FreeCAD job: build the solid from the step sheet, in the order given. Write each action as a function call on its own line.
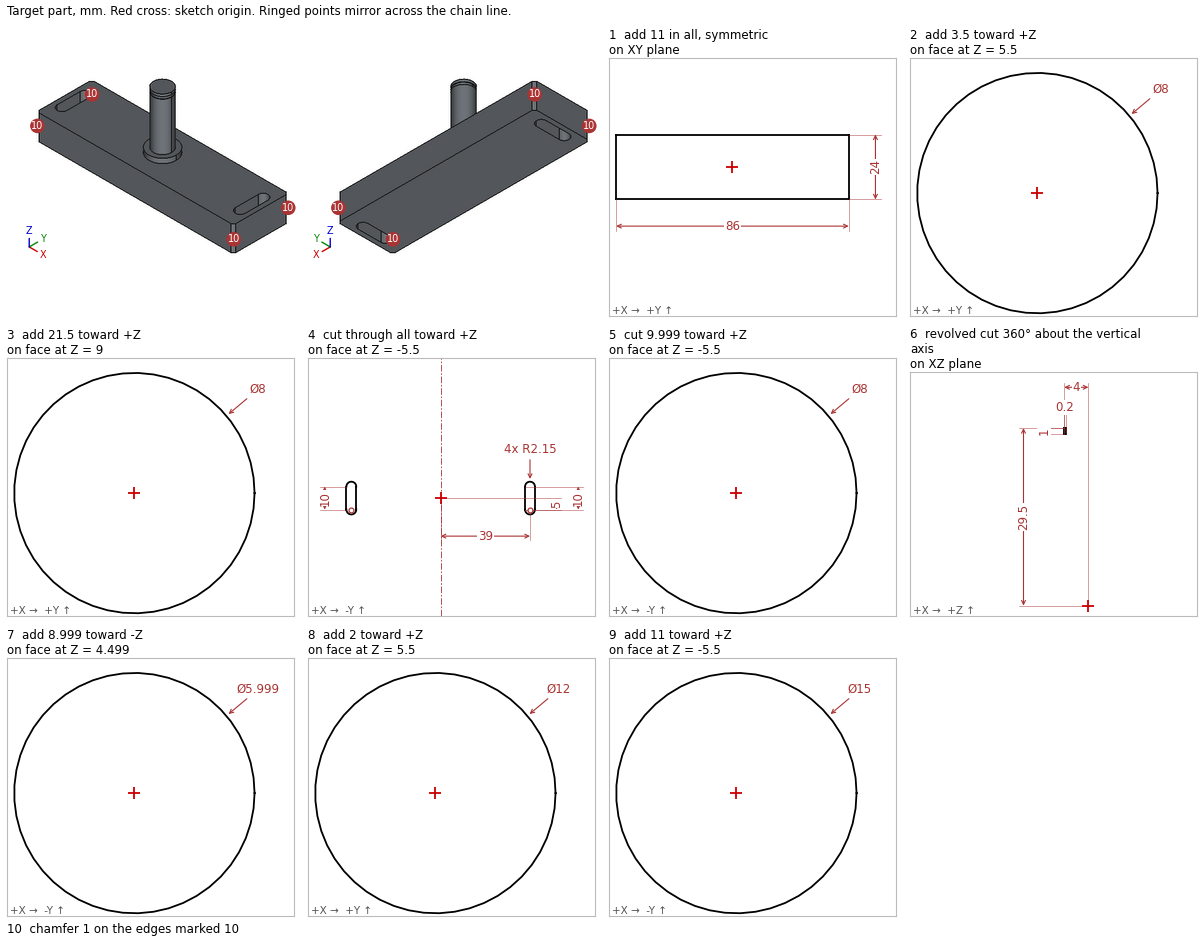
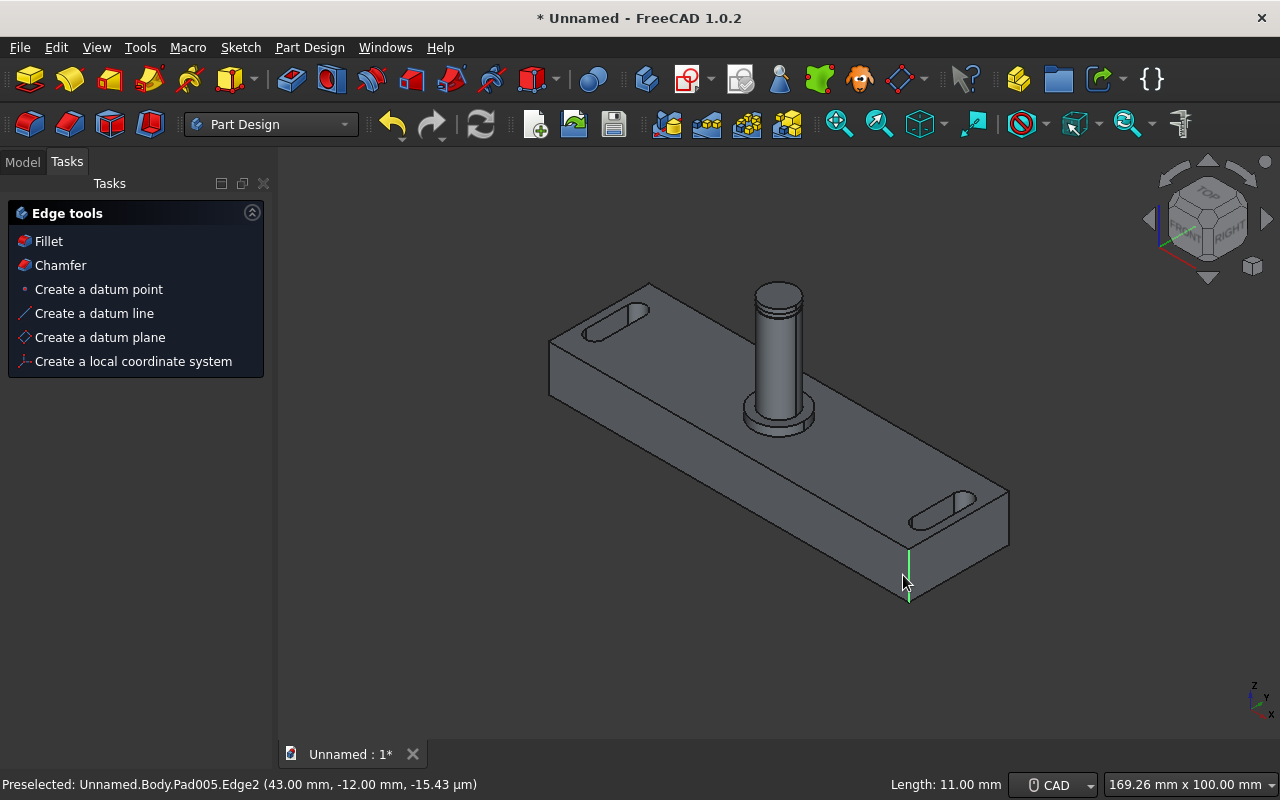
key(2)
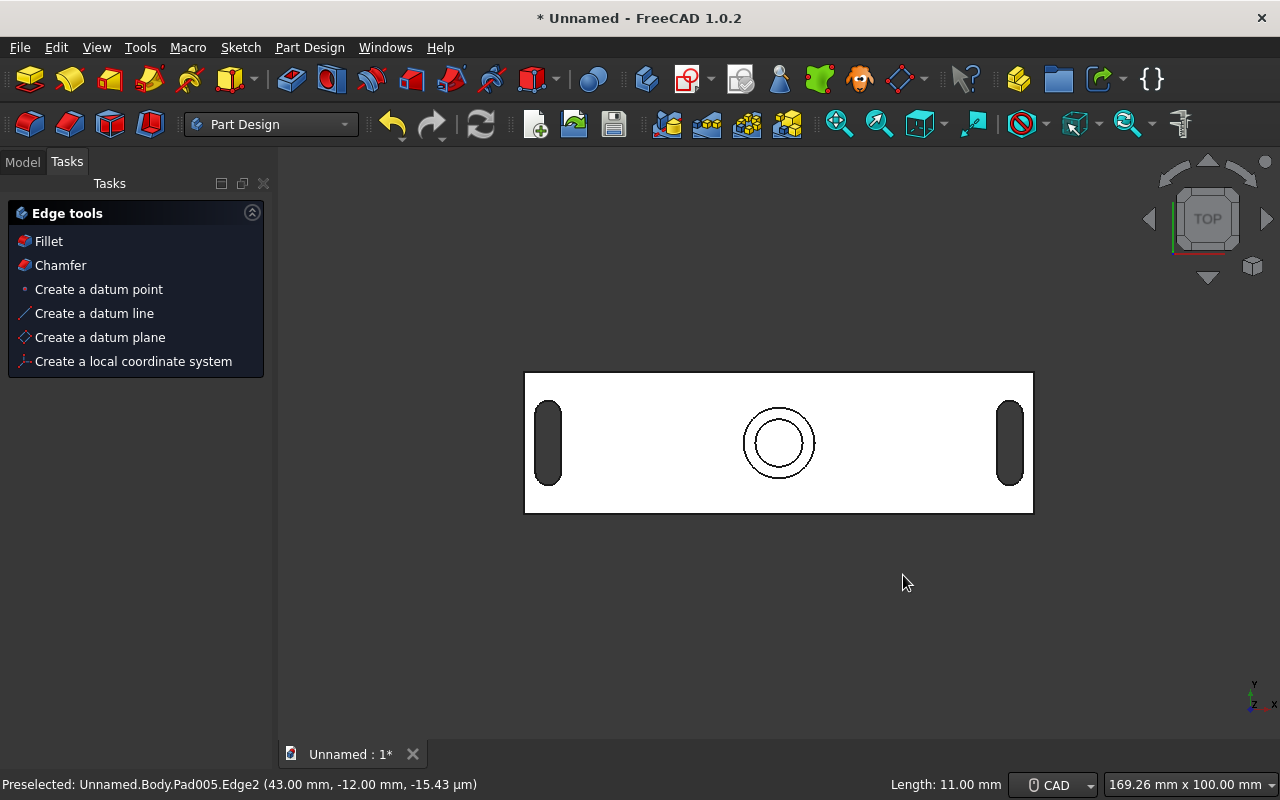
key(1)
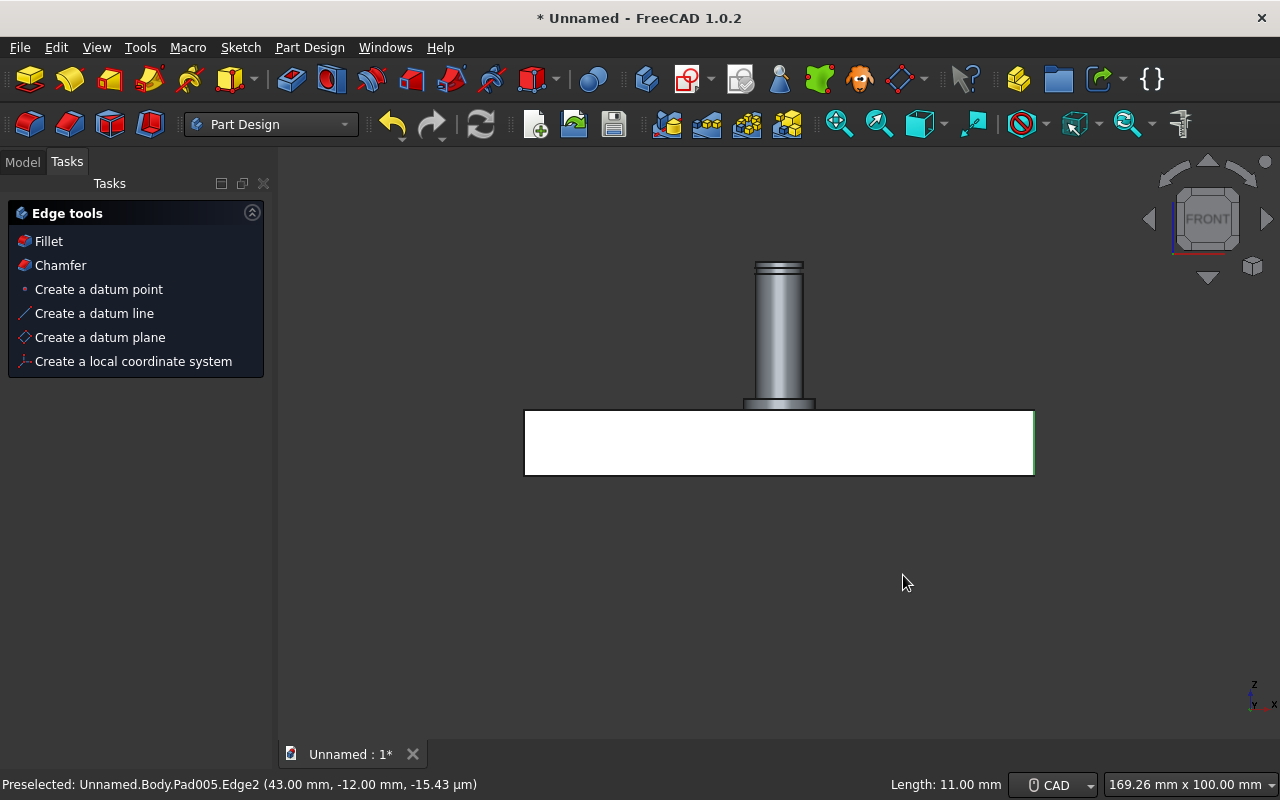
click(524, 442, ctrl)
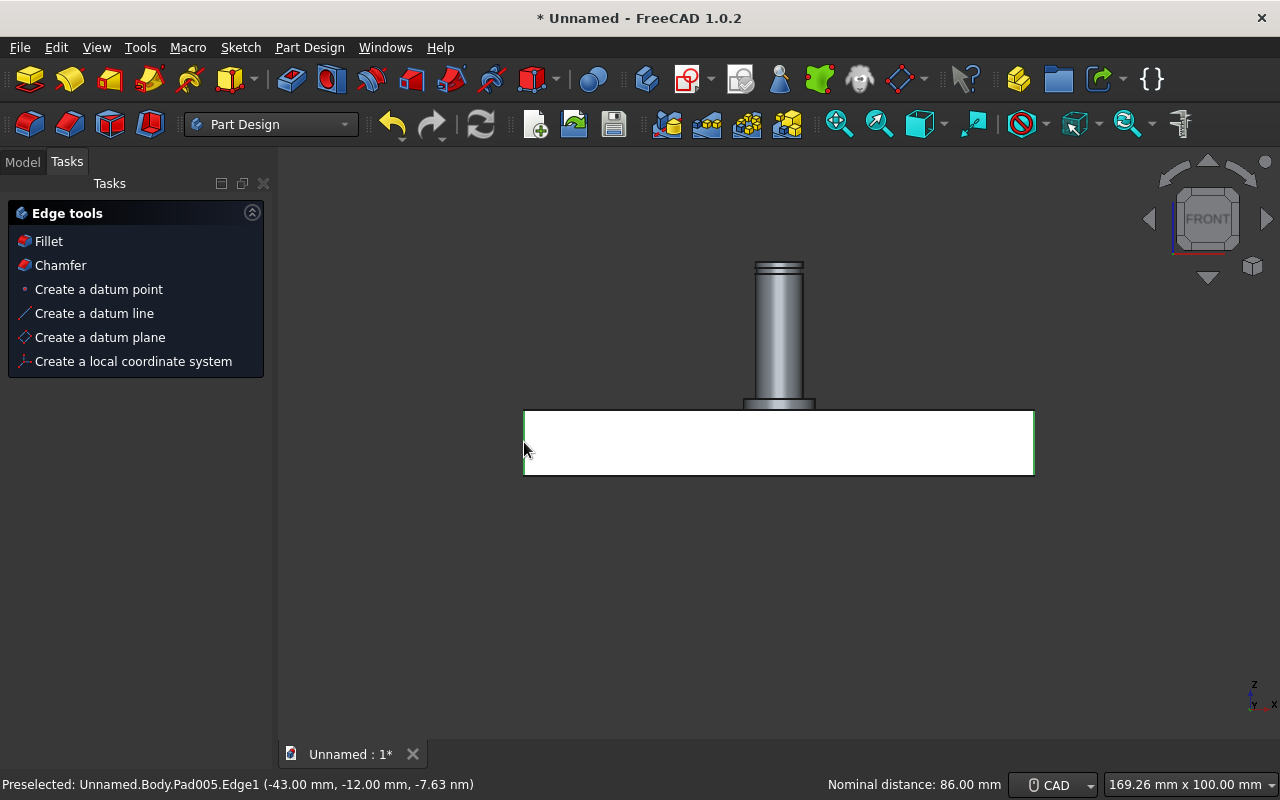
key(3)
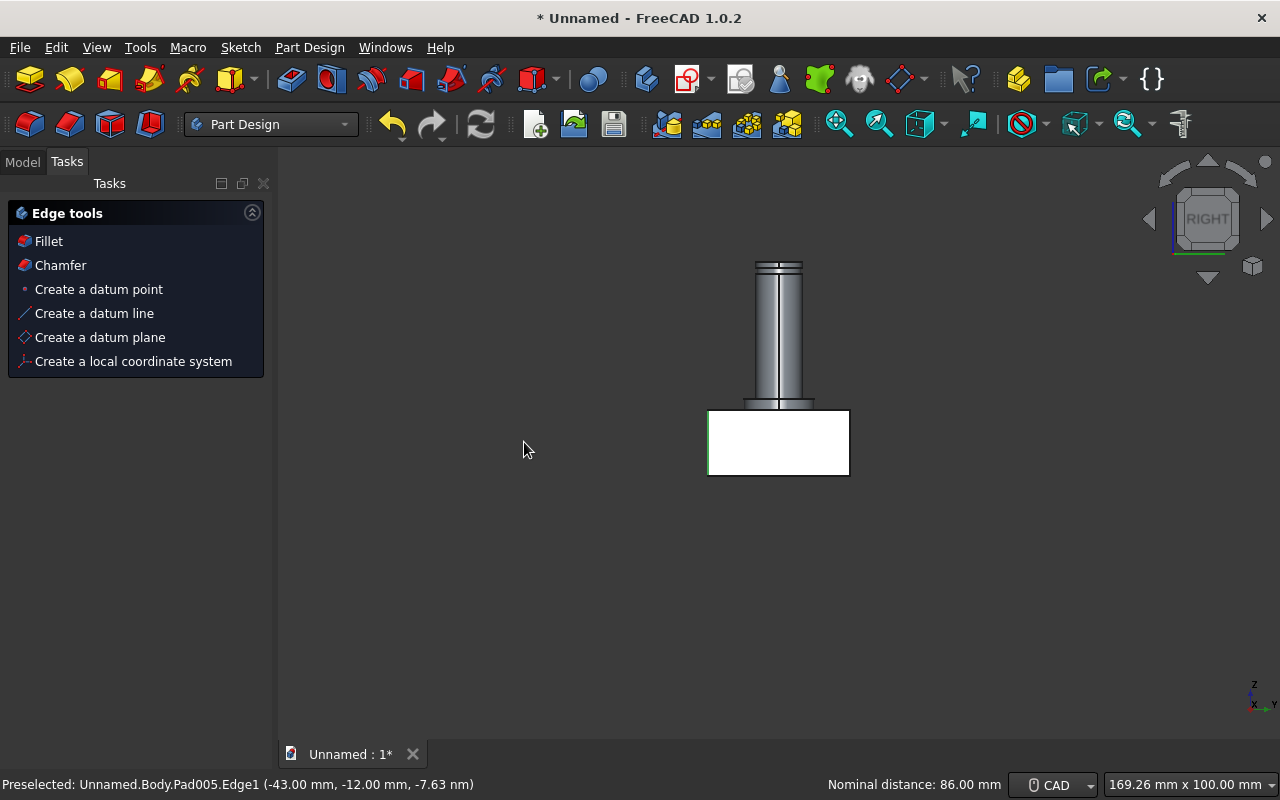
click(840, 124)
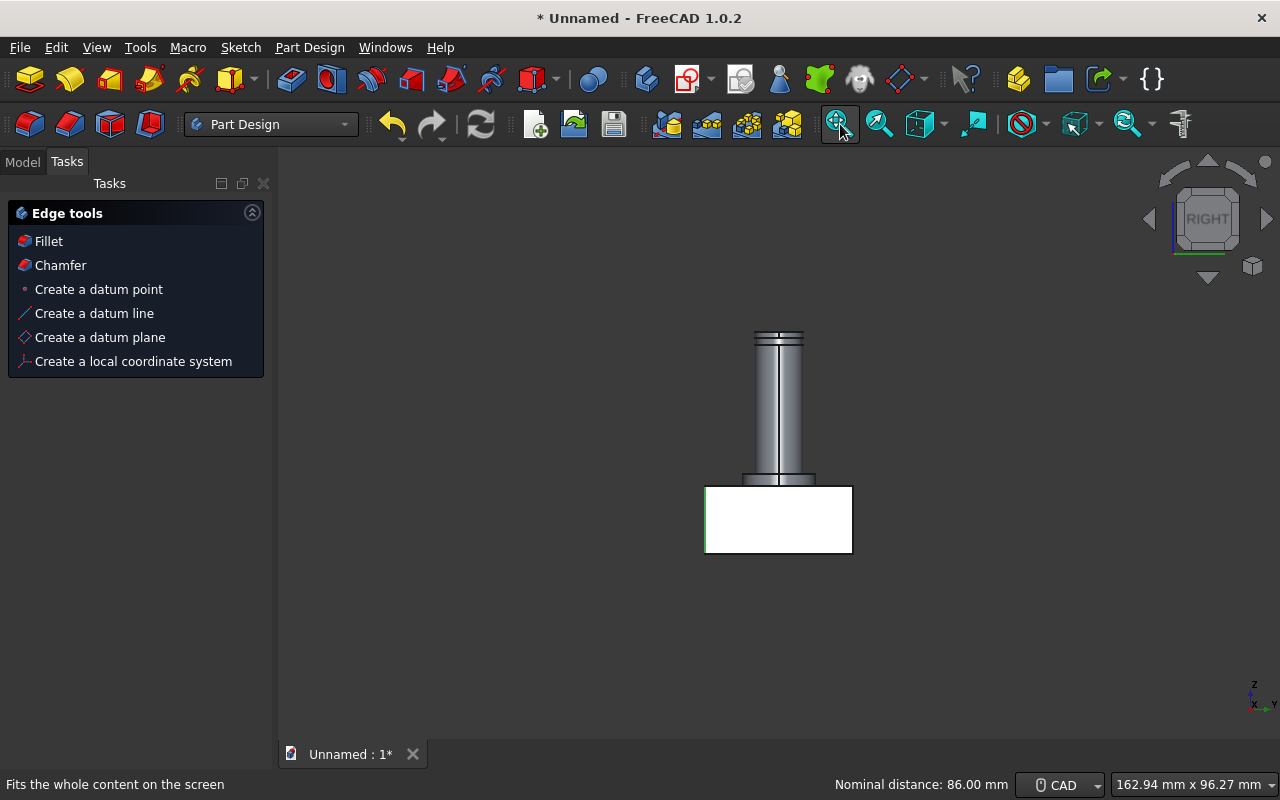
click(853, 519, ctrl)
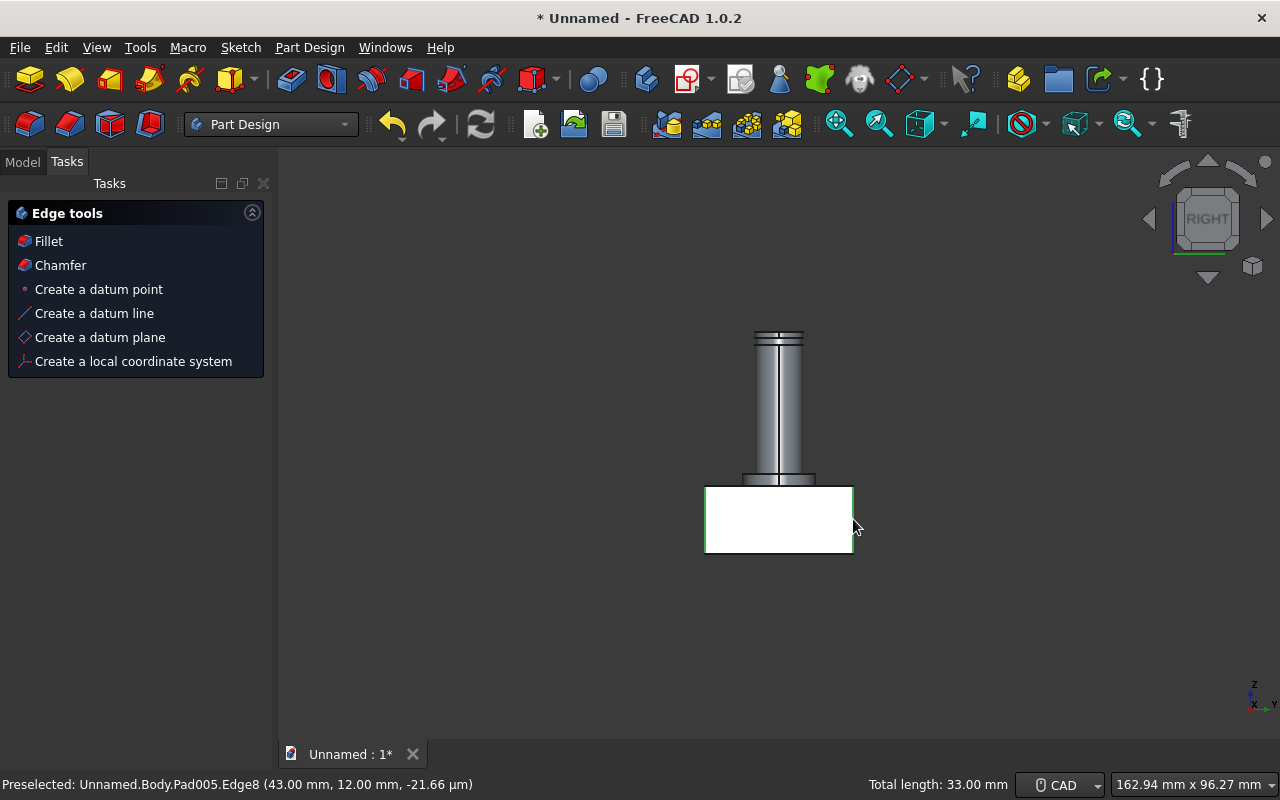
key(5)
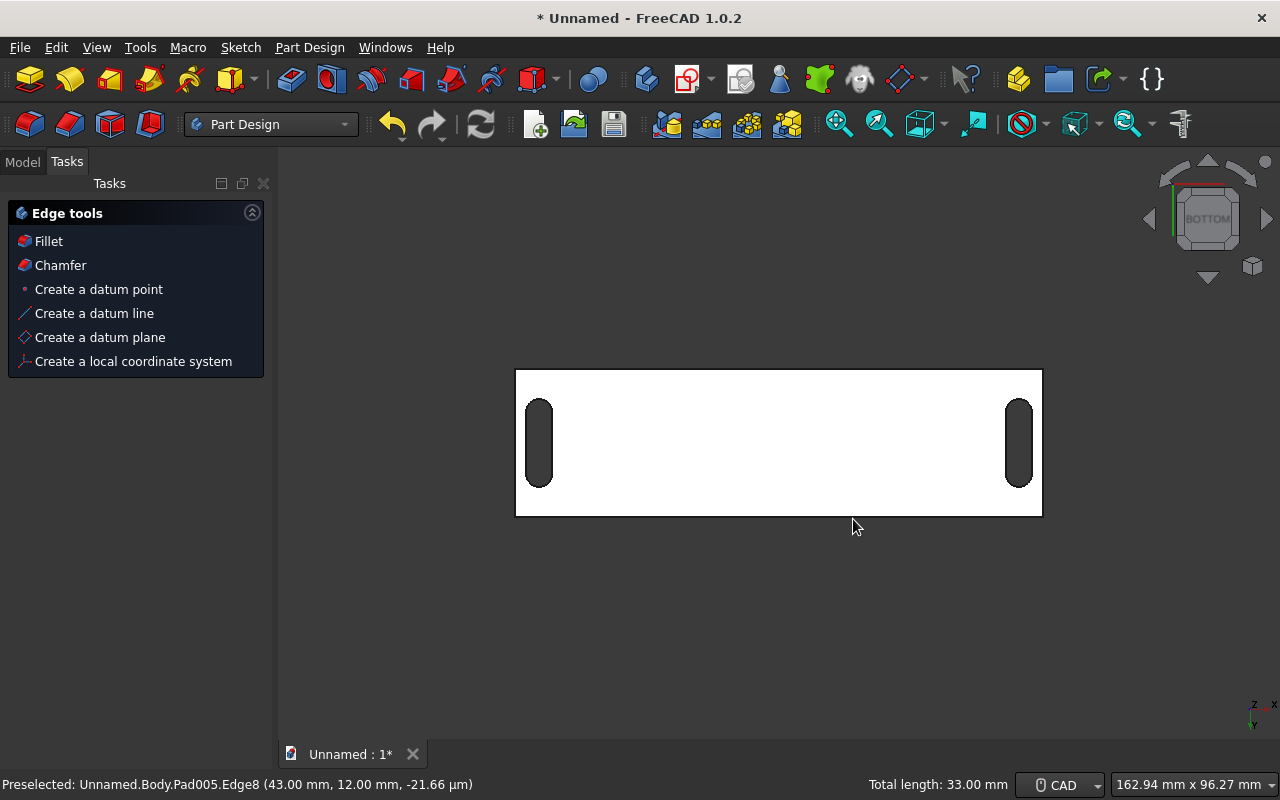
key(4)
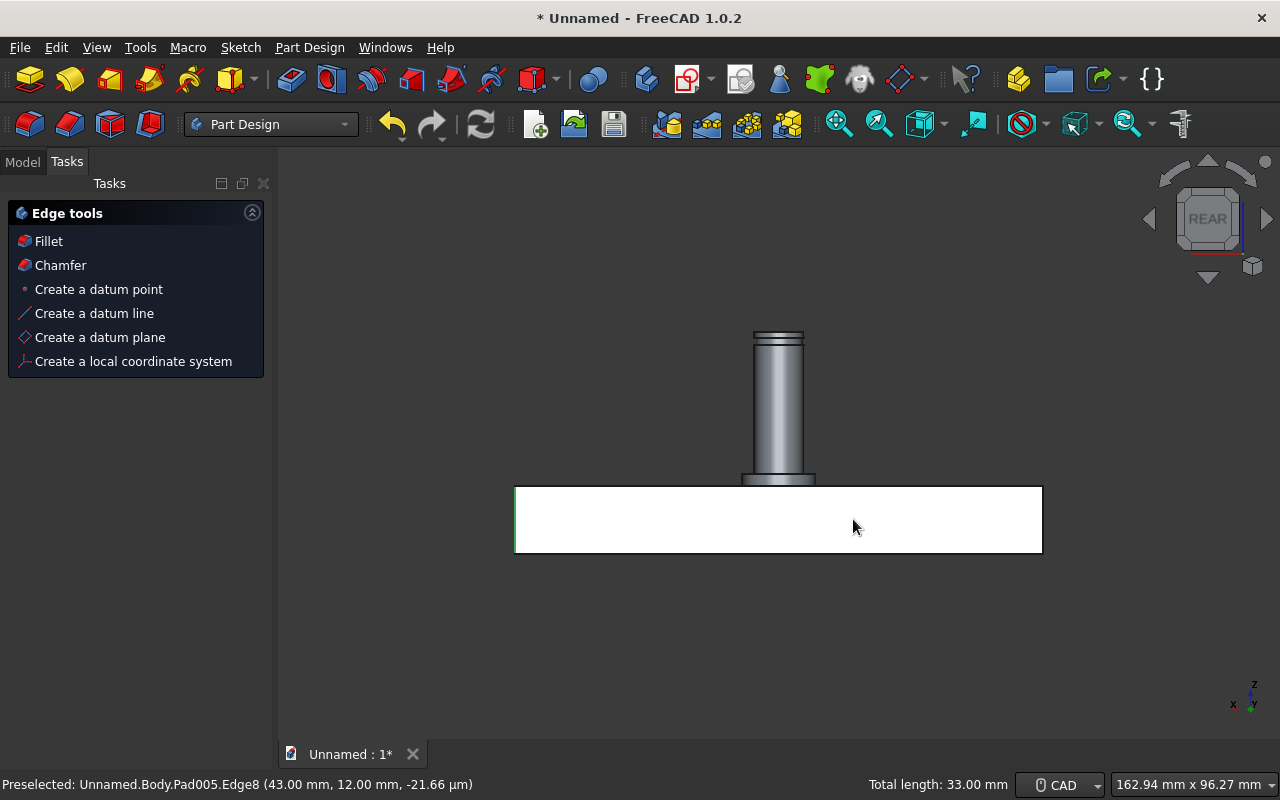
click(1043, 519, ctrl)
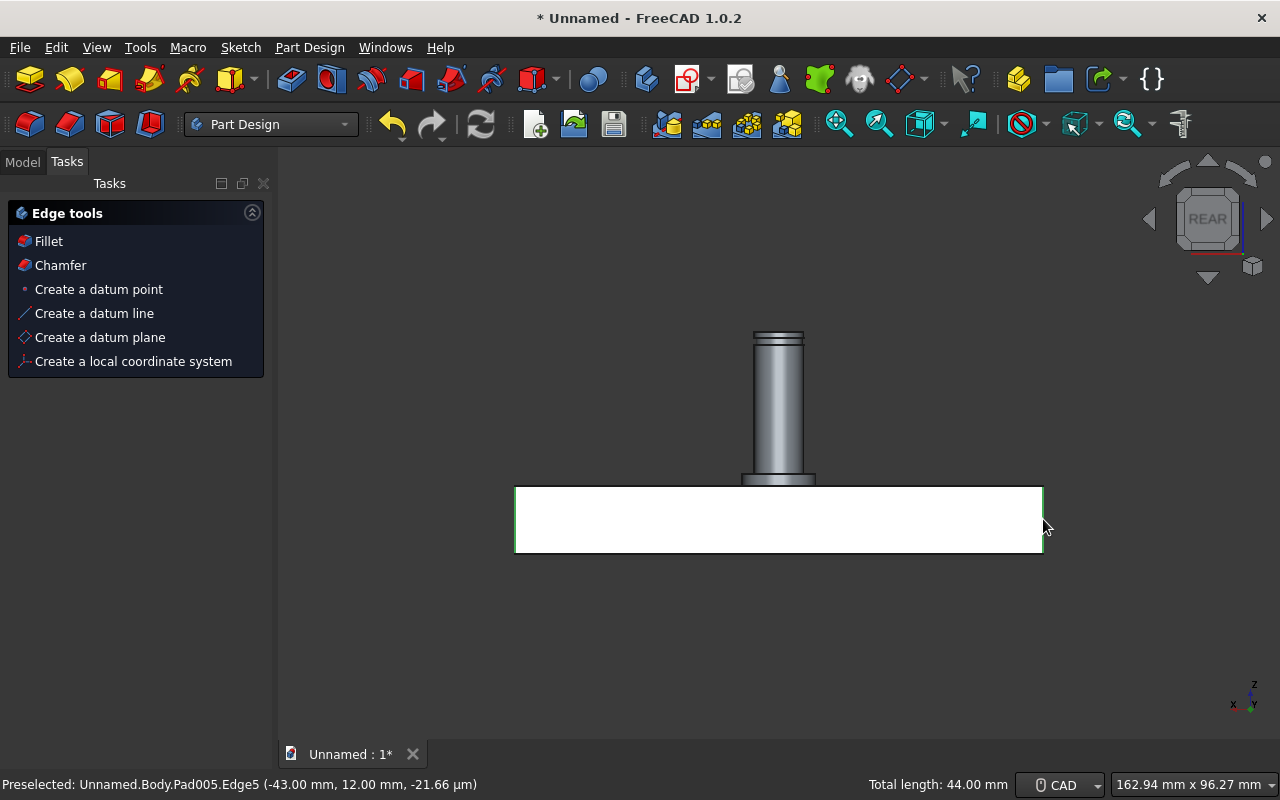
click(70, 124)